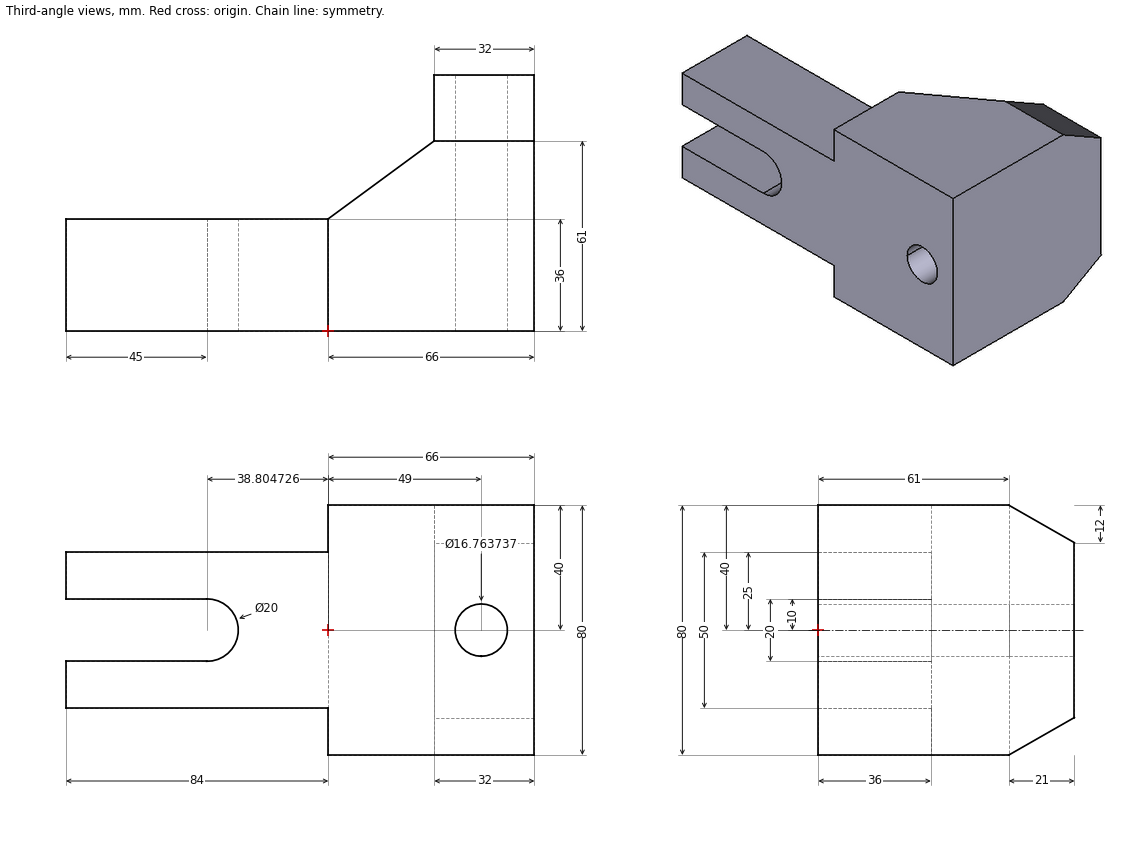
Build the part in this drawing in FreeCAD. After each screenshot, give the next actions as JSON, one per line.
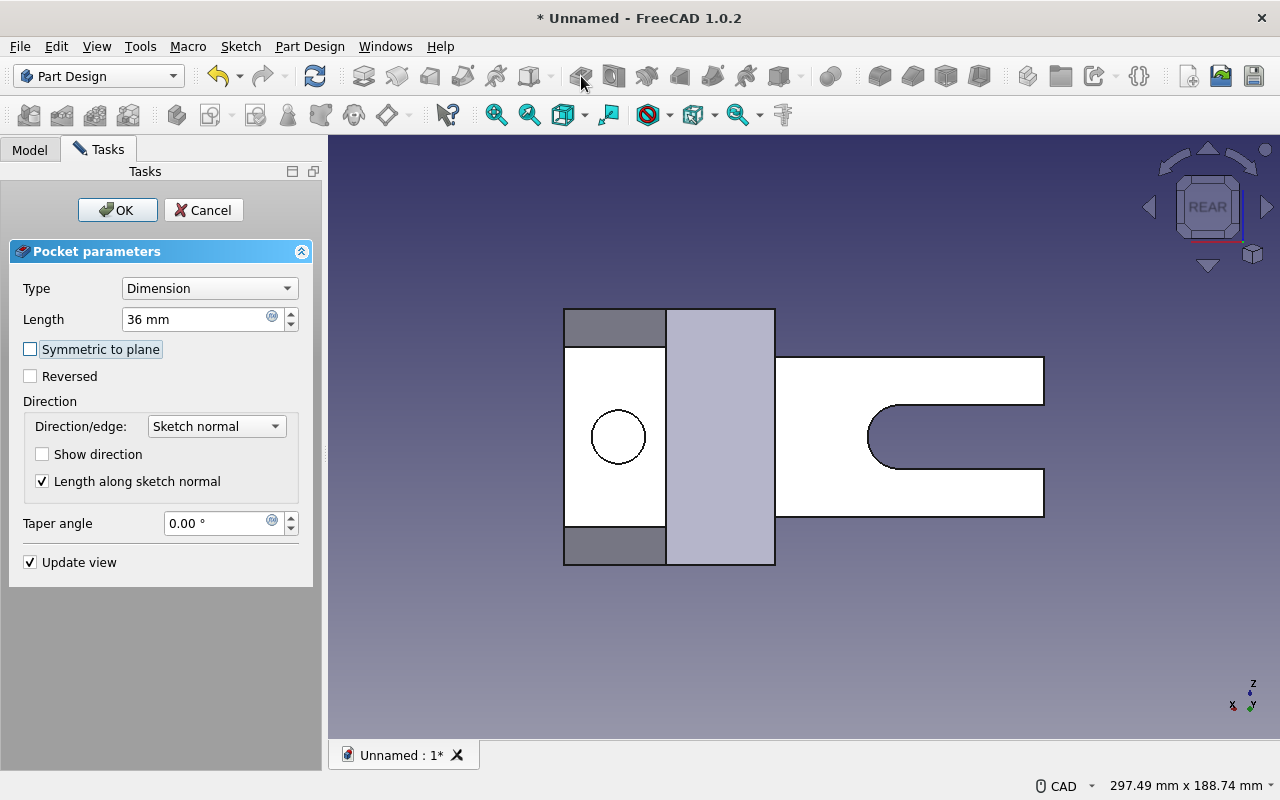
{"action": "left_click", "coordinate": [118, 210]}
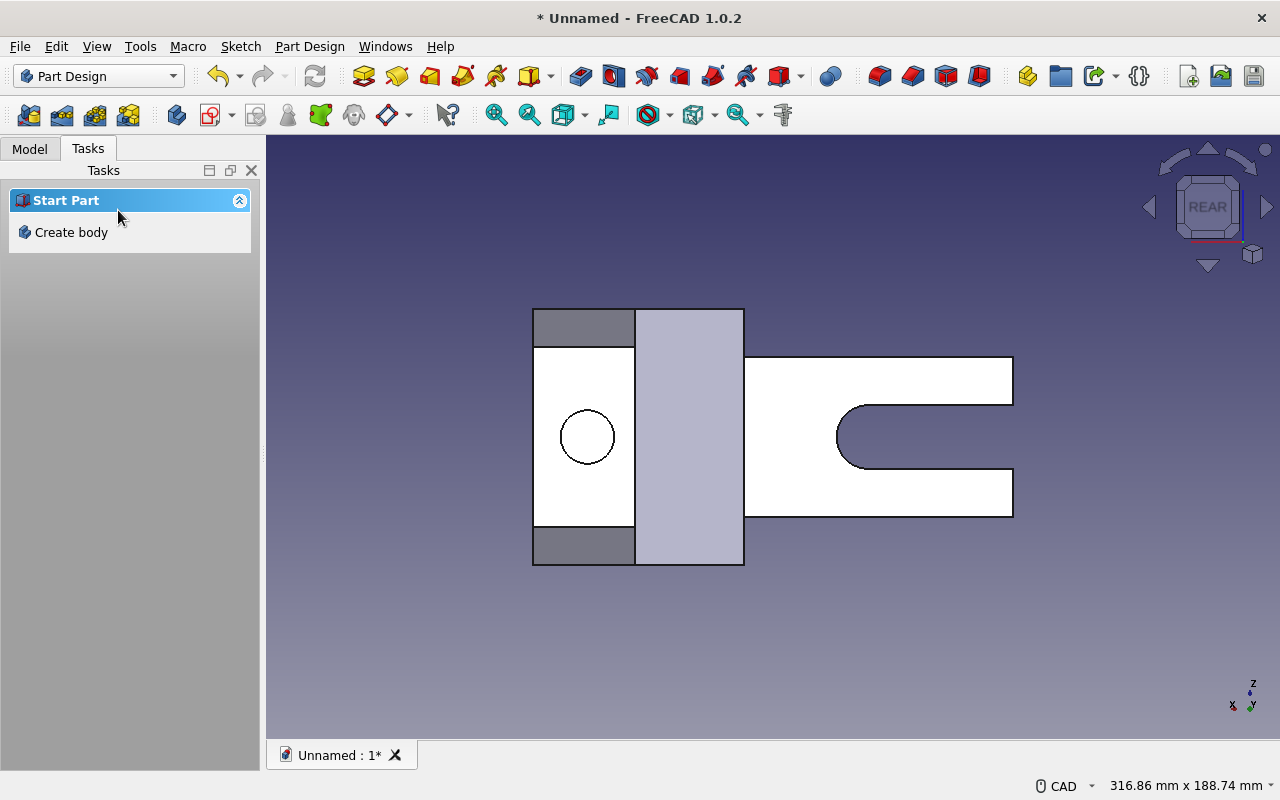
{"action": "left_click", "coordinate": [570, 385]}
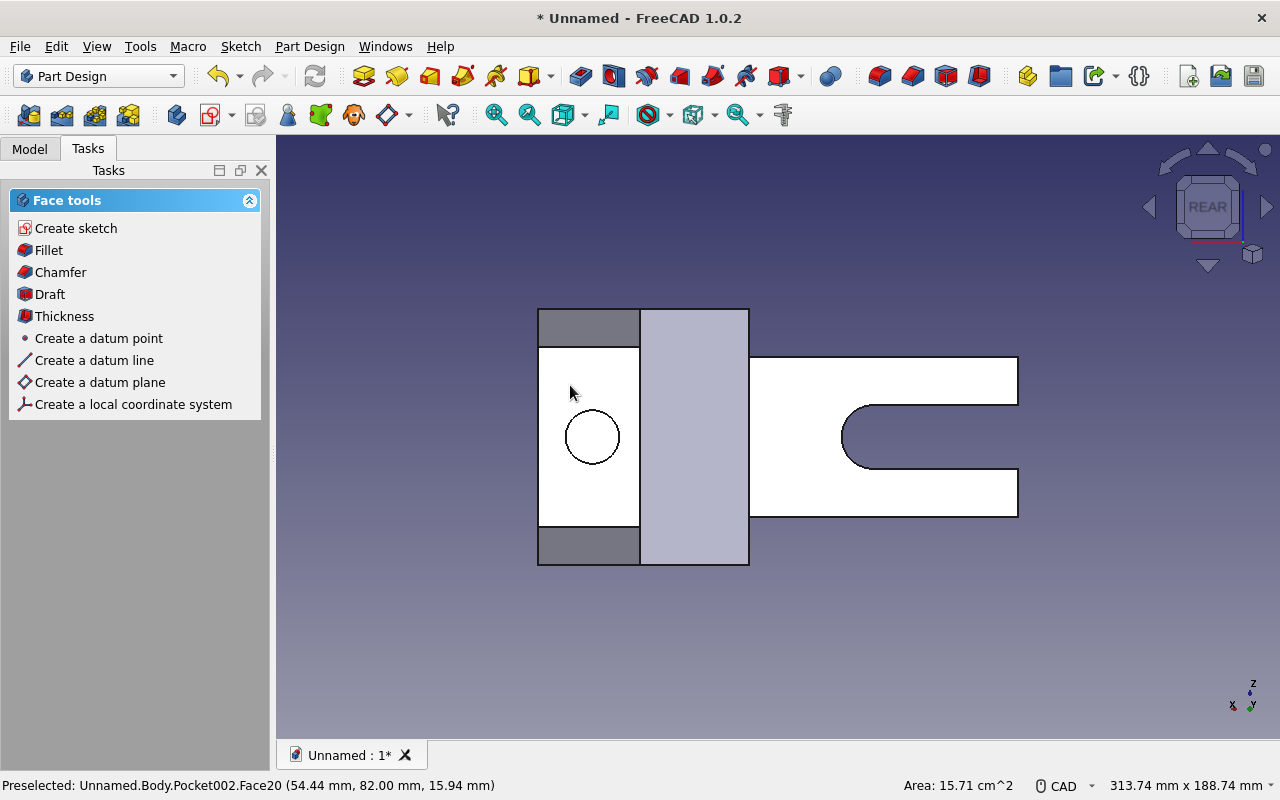
{"action": "left_click", "coordinate": [210, 116]}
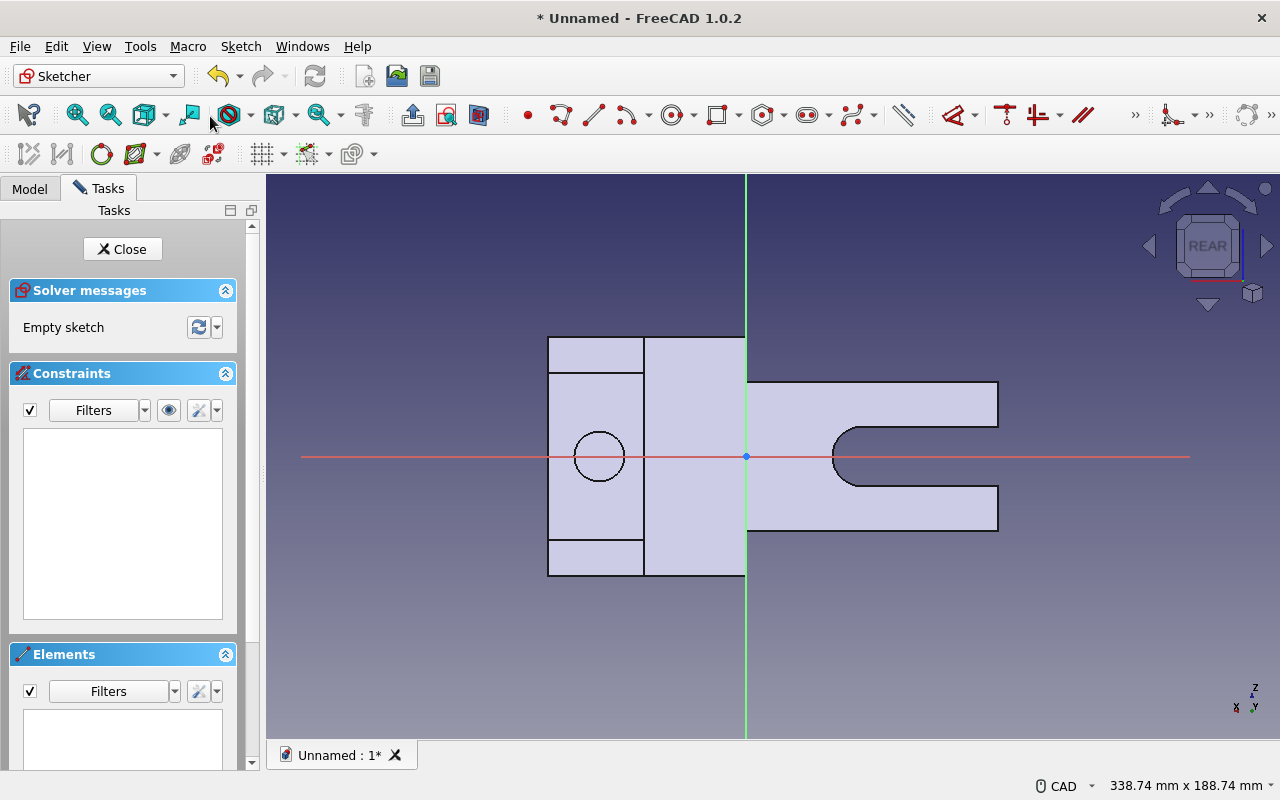
{"action": "scroll", "coordinate": [583, 457], "scroll_direction": "up", "scroll_amount": 10}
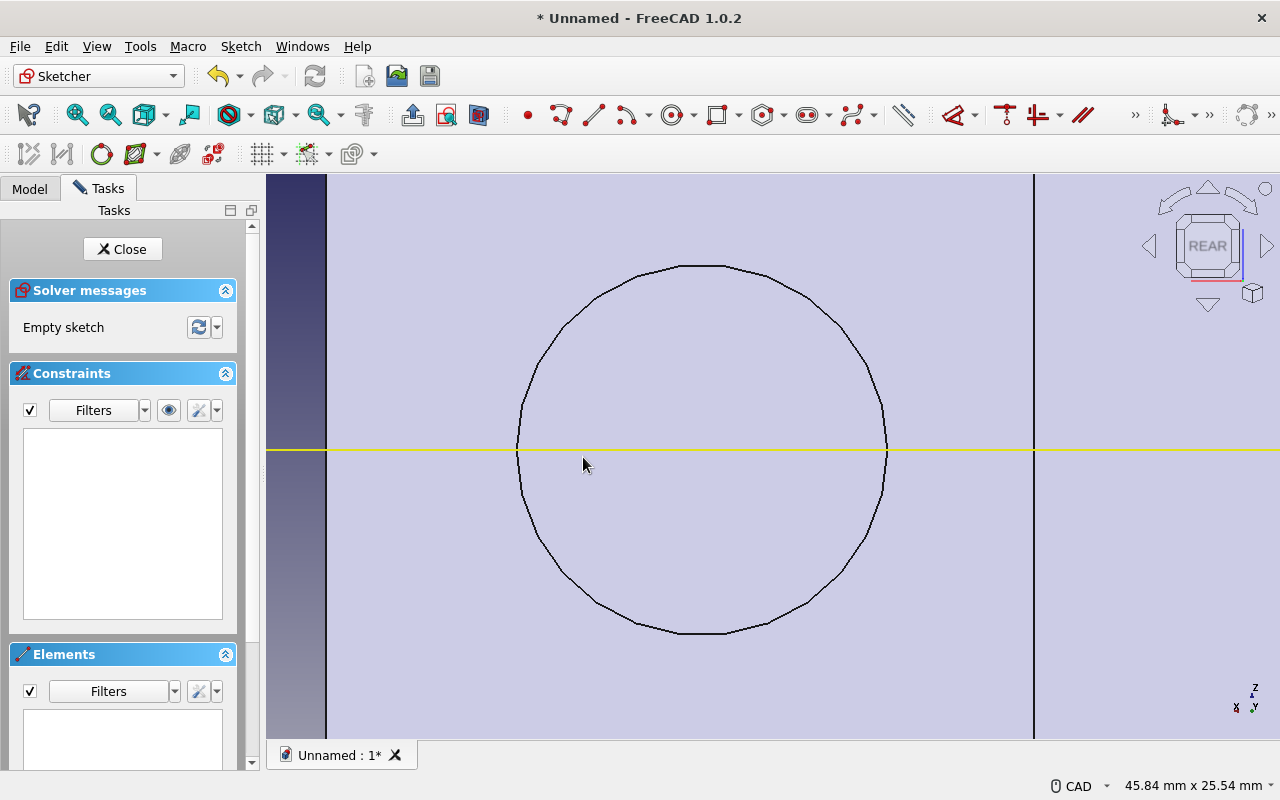
{"action": "key", "text": "g c"}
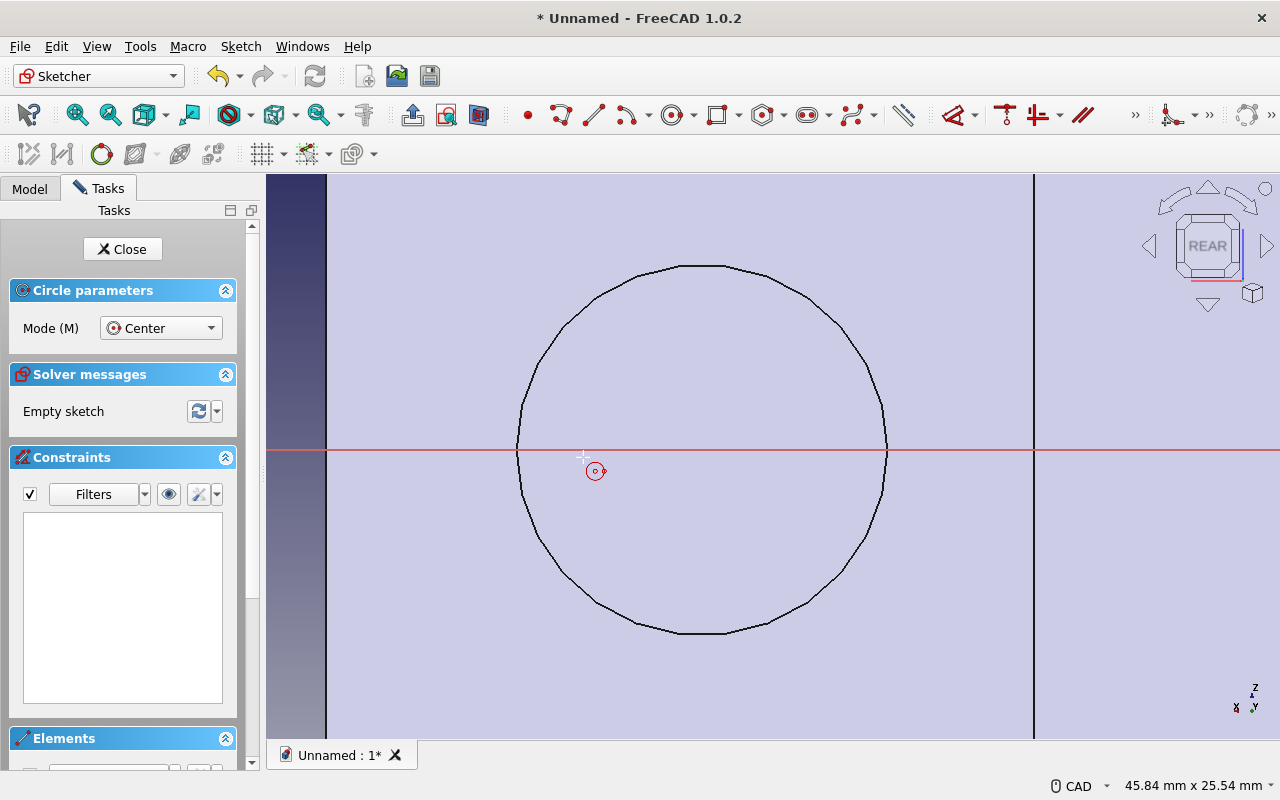
{"action": "left_click", "coordinate": [702, 450]}
{"action": "left_click", "coordinate": [833, 319]}
{"action": "key", "text": "Escape"}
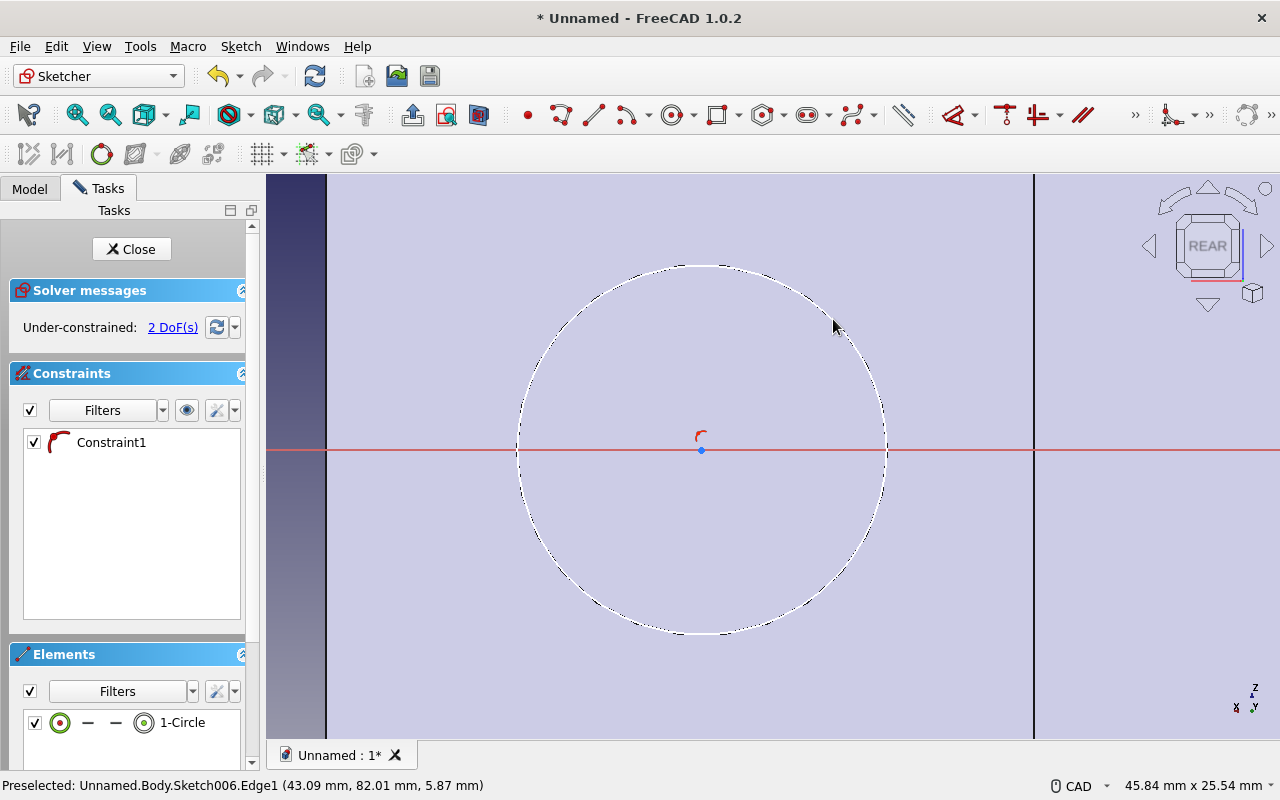
{"action": "left_click", "coordinate": [952, 116]}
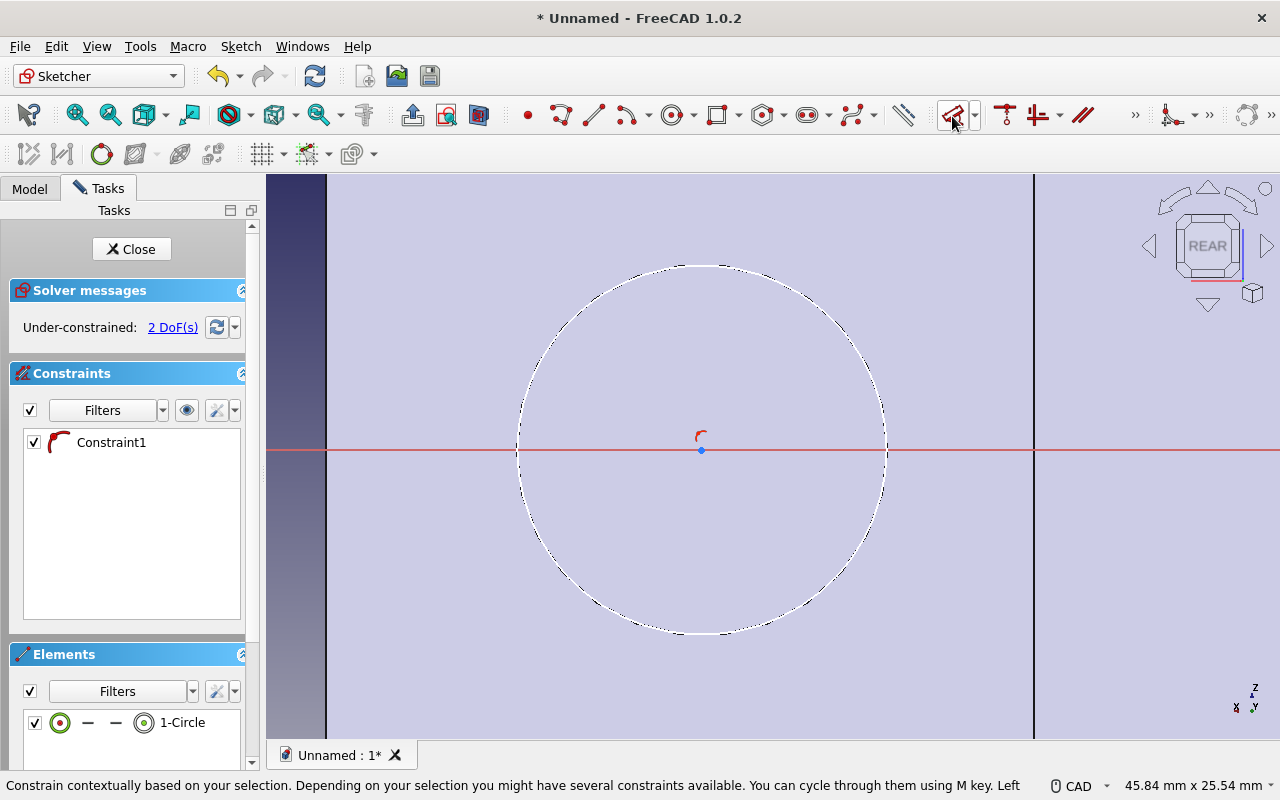
{"action": "left_click", "coordinate": [832, 319]}
{"action": "left_click", "coordinate": [855, 296]}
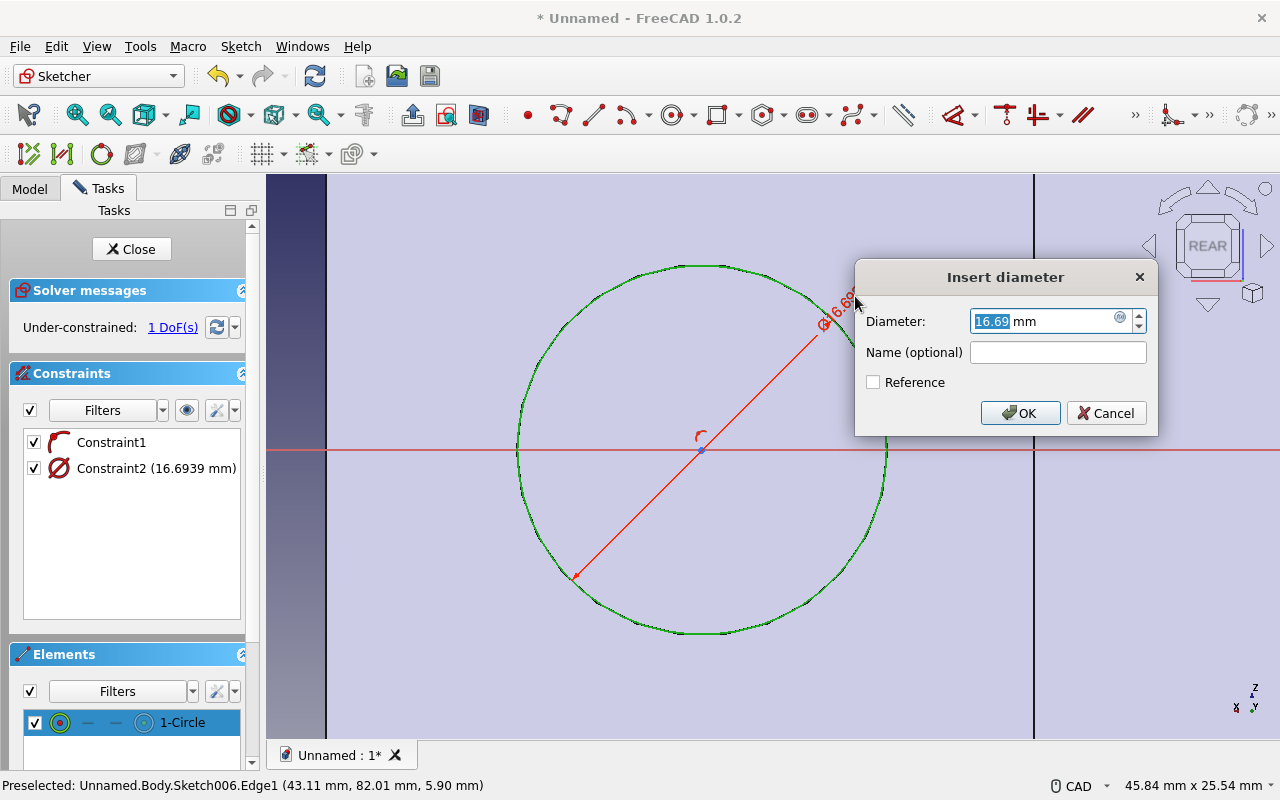
{"action": "type", "text": "16.763737"}
{"action": "key", "text": "Return"}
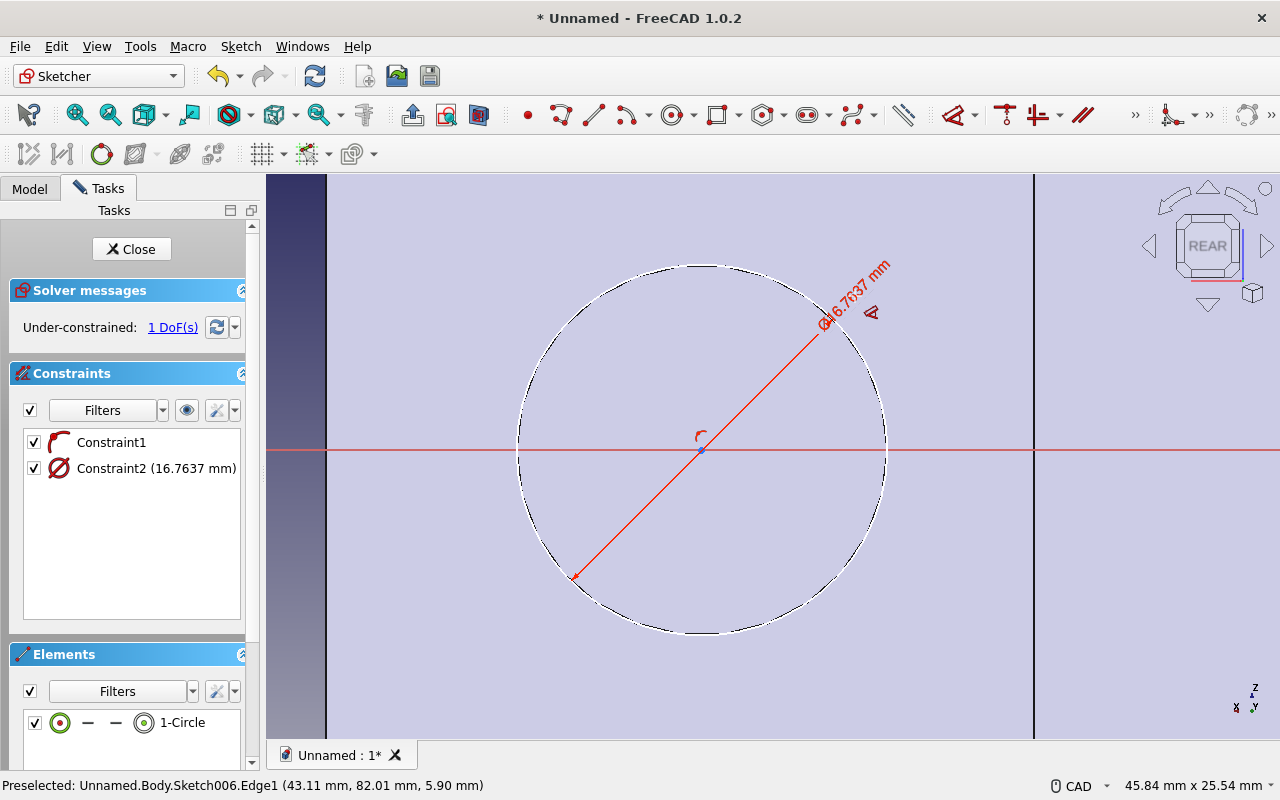
{"action": "left_click", "coordinate": [702, 450]}
{"action": "left_click", "coordinate": [908, 484]}